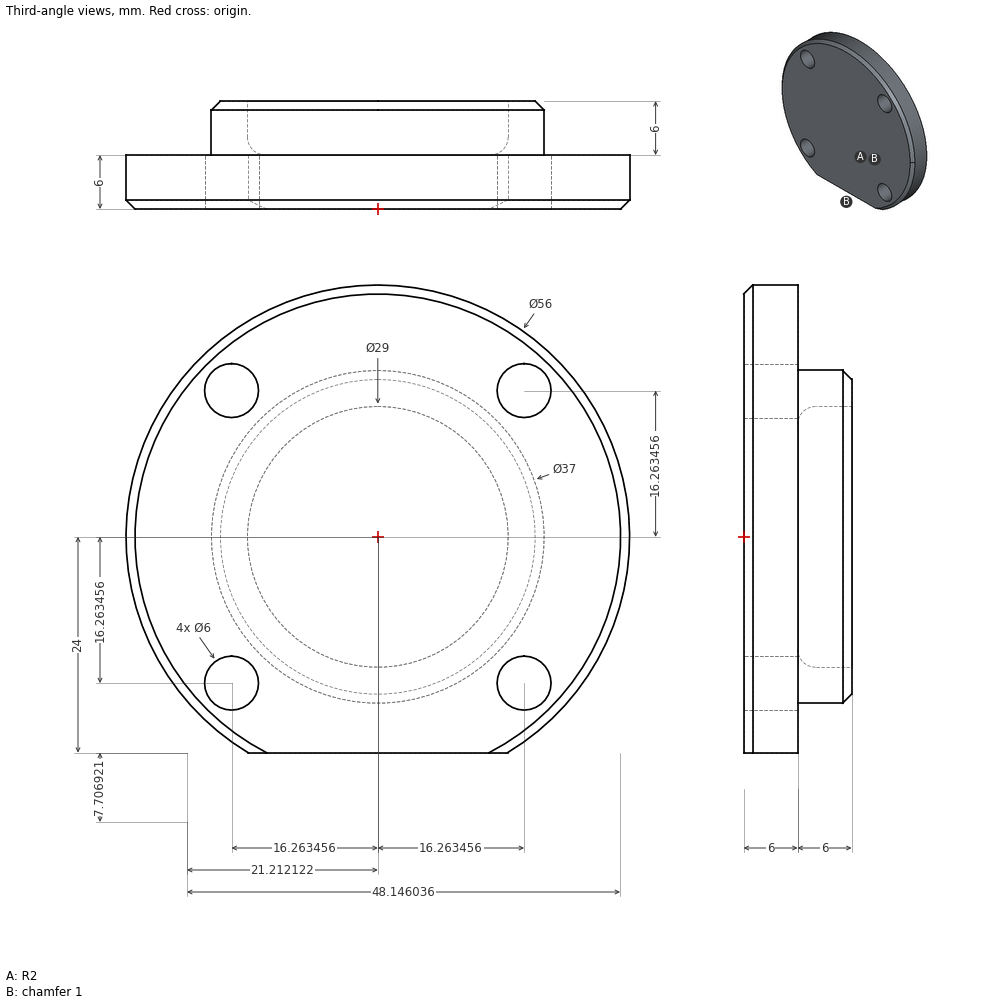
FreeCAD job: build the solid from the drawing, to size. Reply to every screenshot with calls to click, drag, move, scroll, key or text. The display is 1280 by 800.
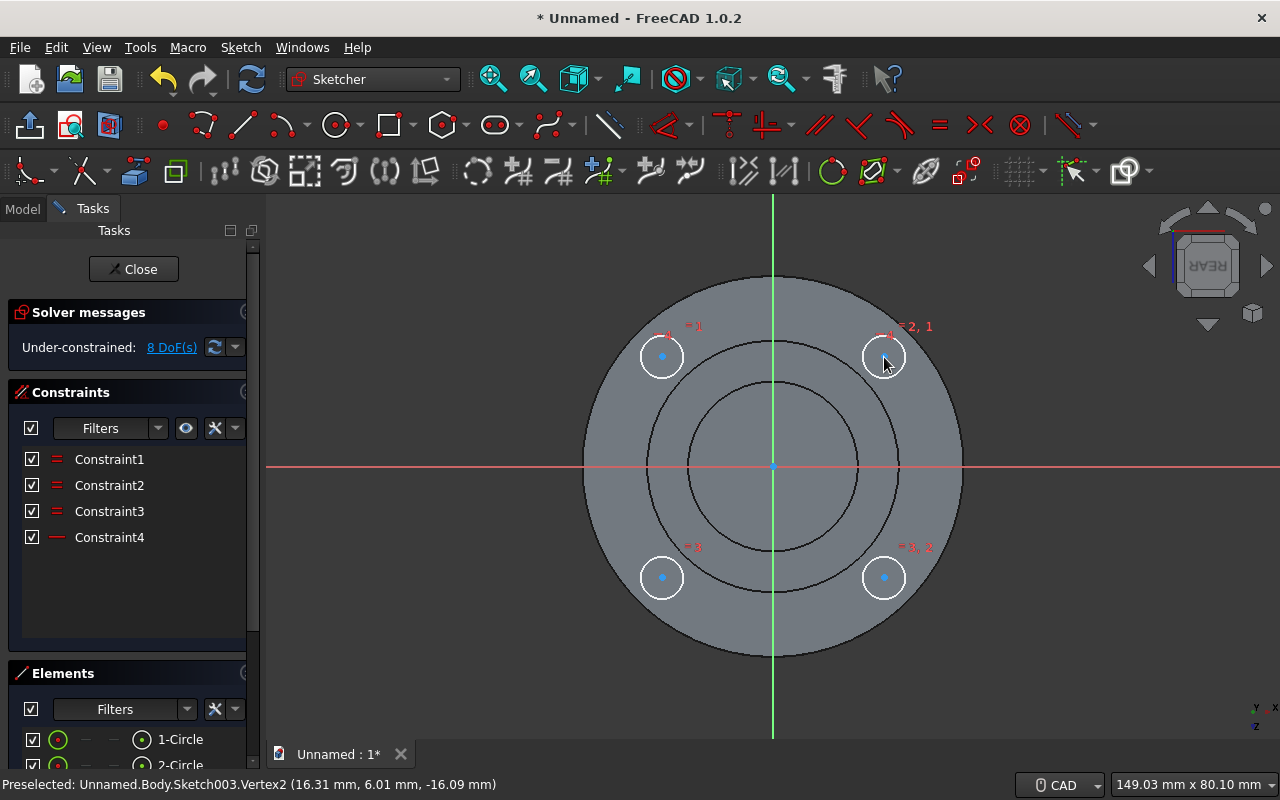
click(884, 357)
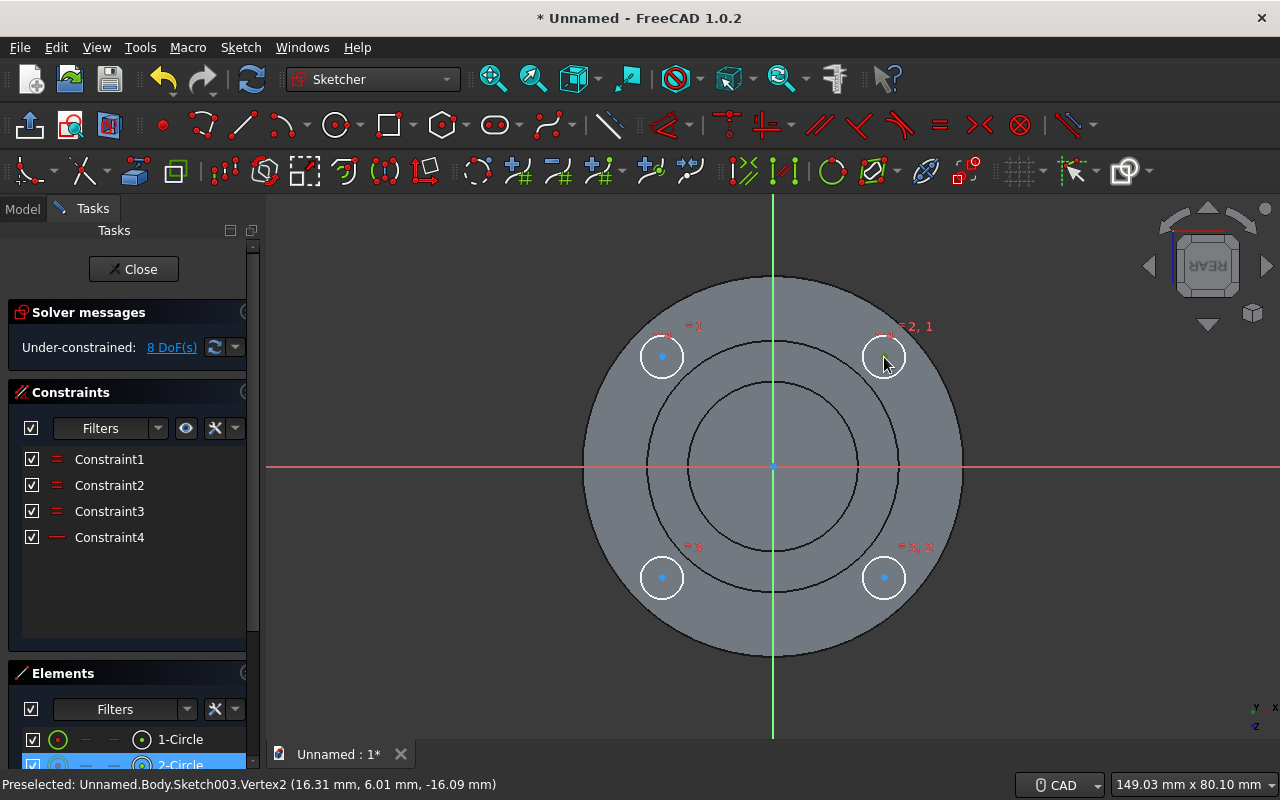
click(884, 578)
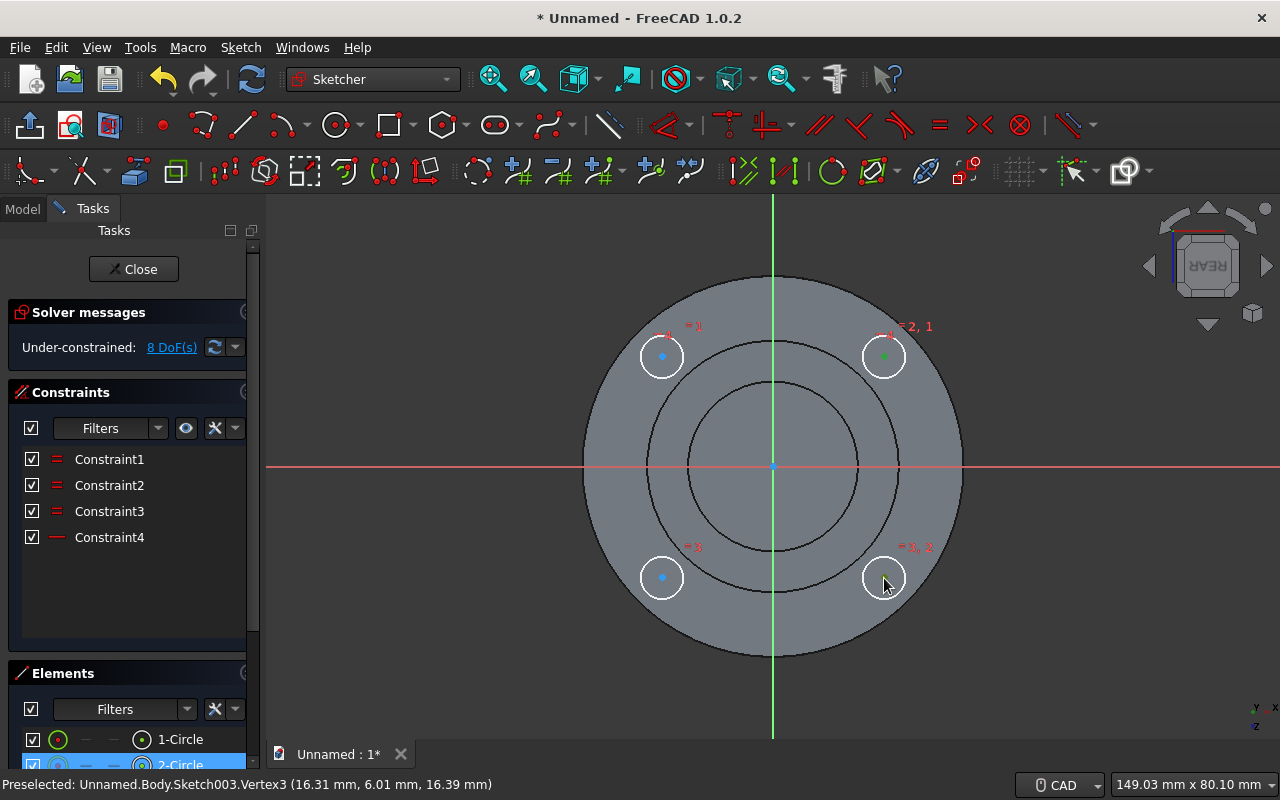
key(v)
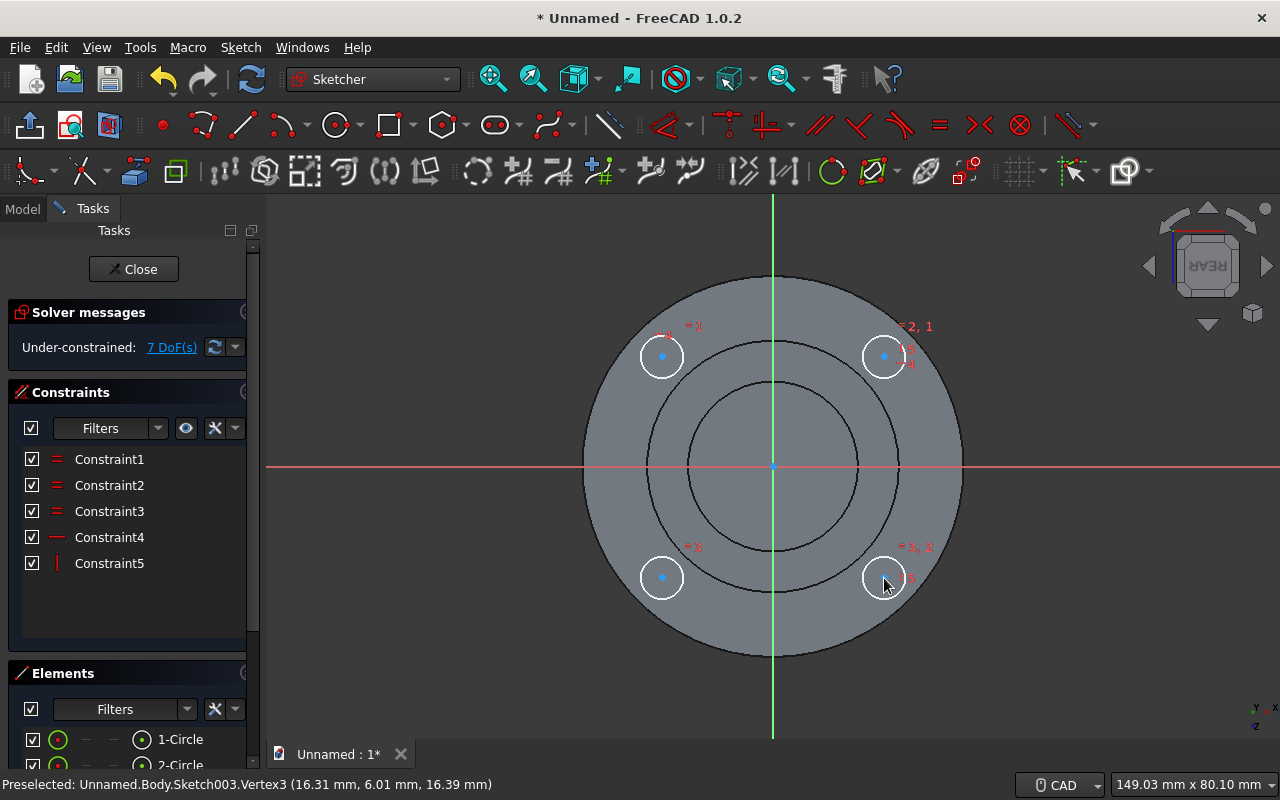
click(662, 357)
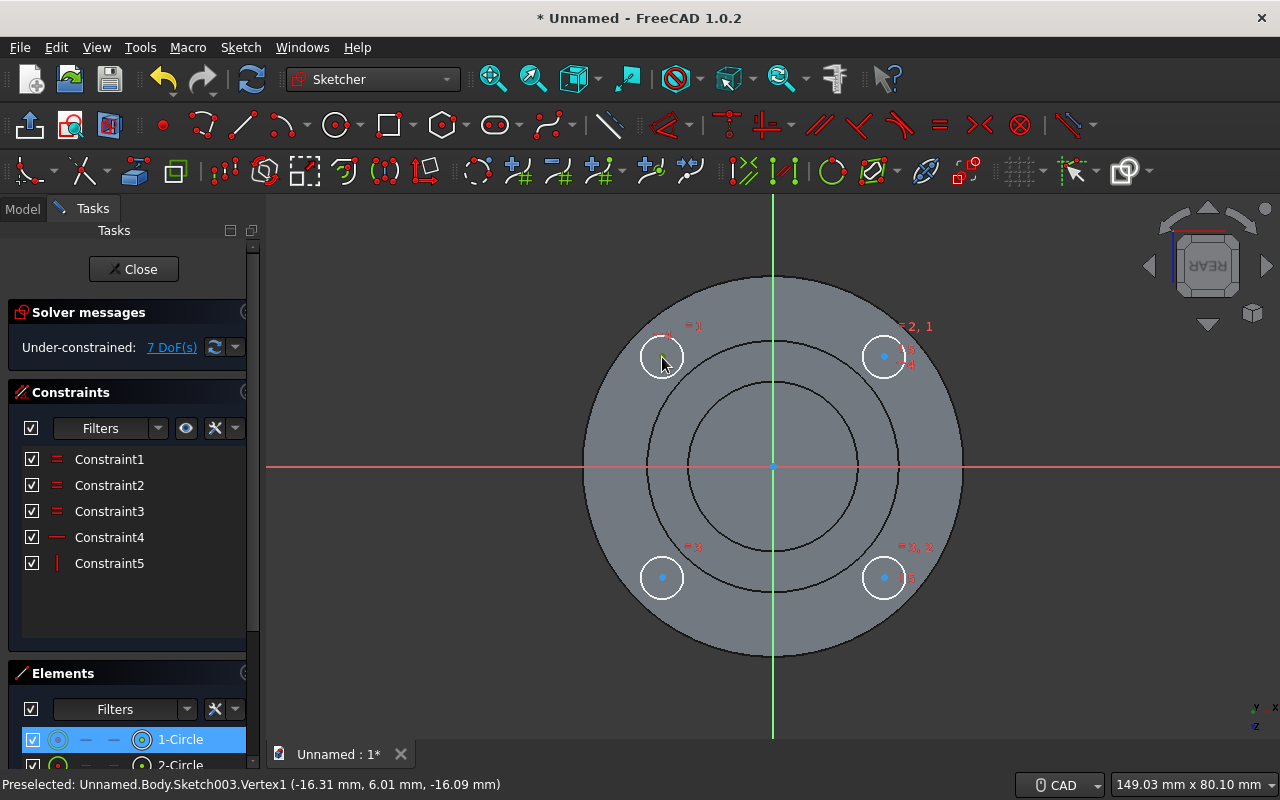
click(662, 578)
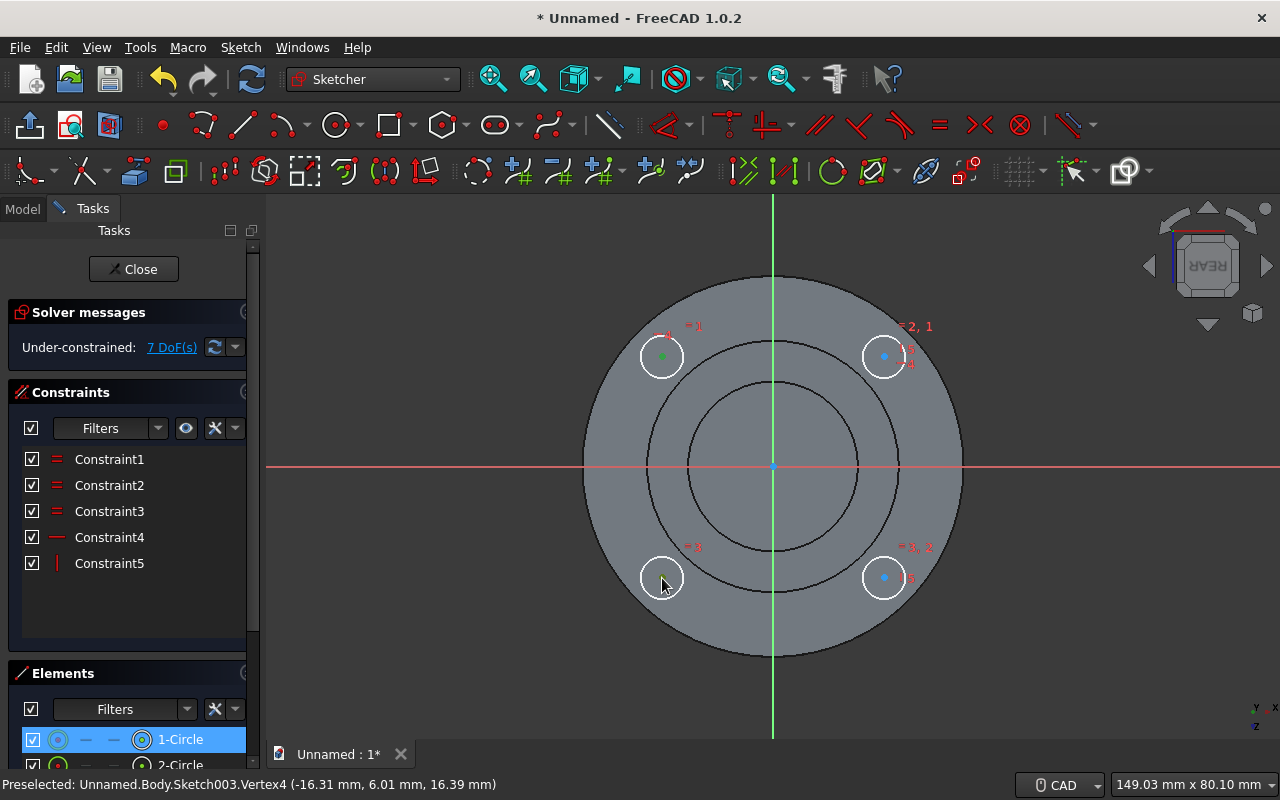
key(v)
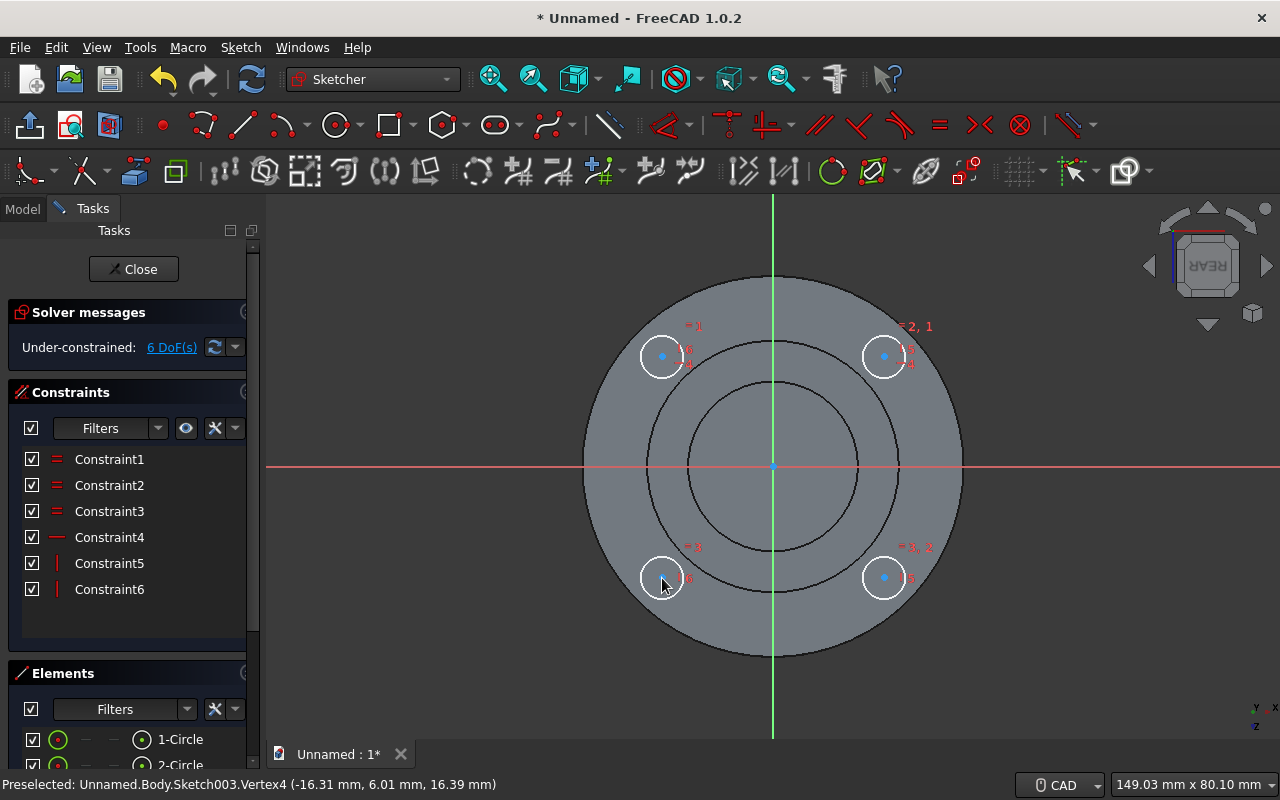
click(884, 578)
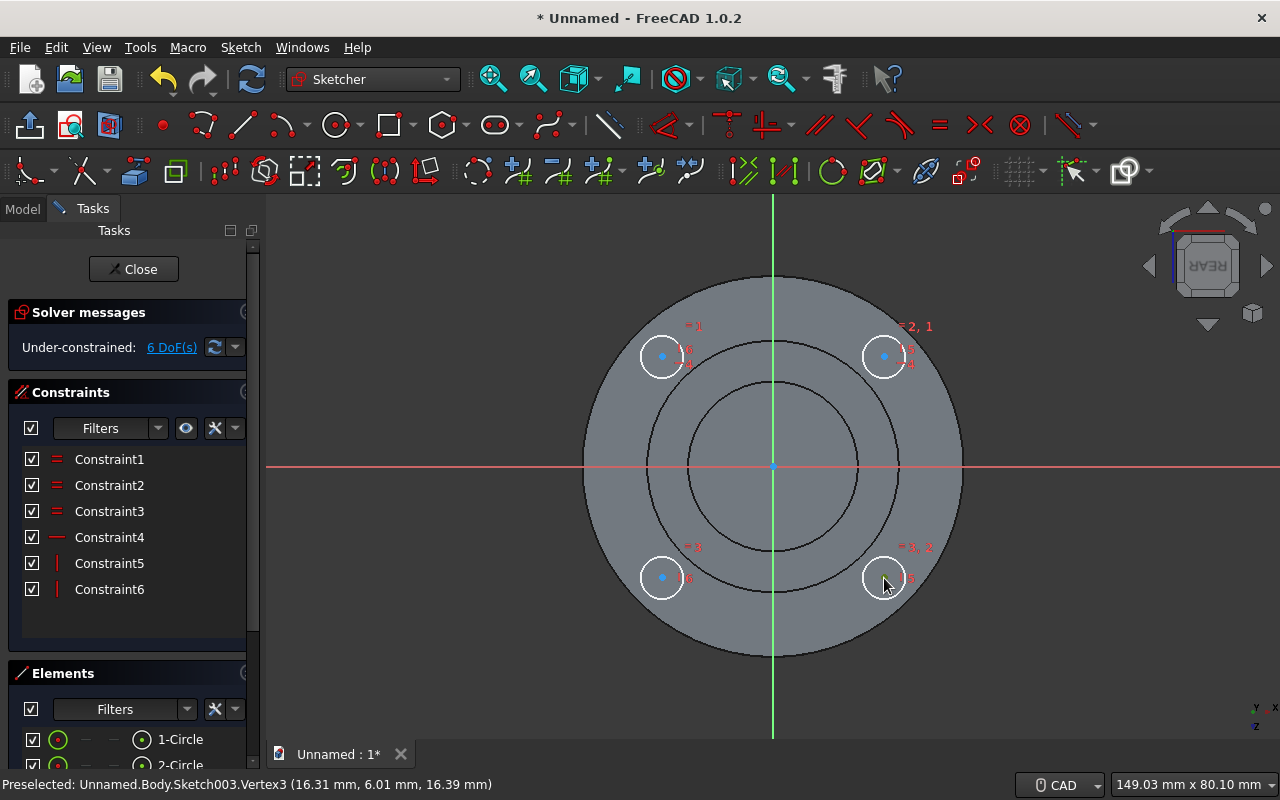
click(662, 578)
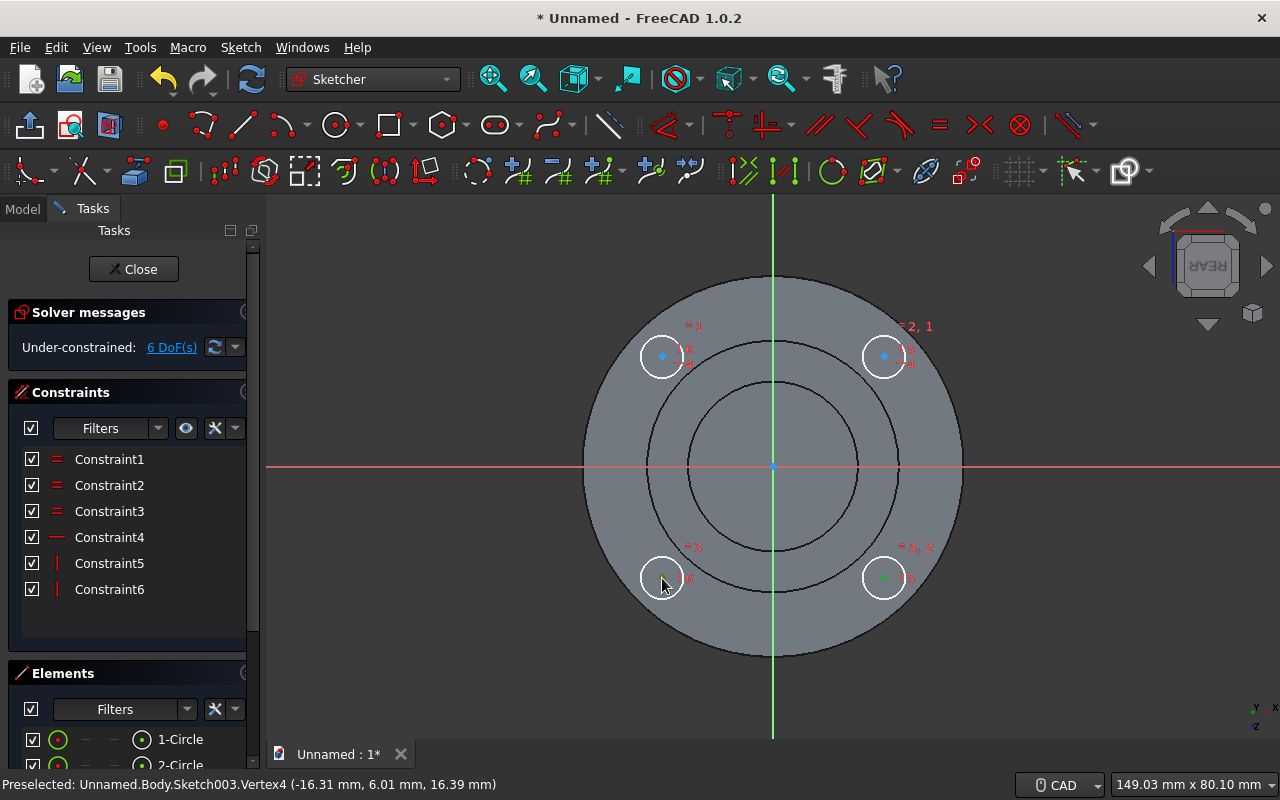
key(h)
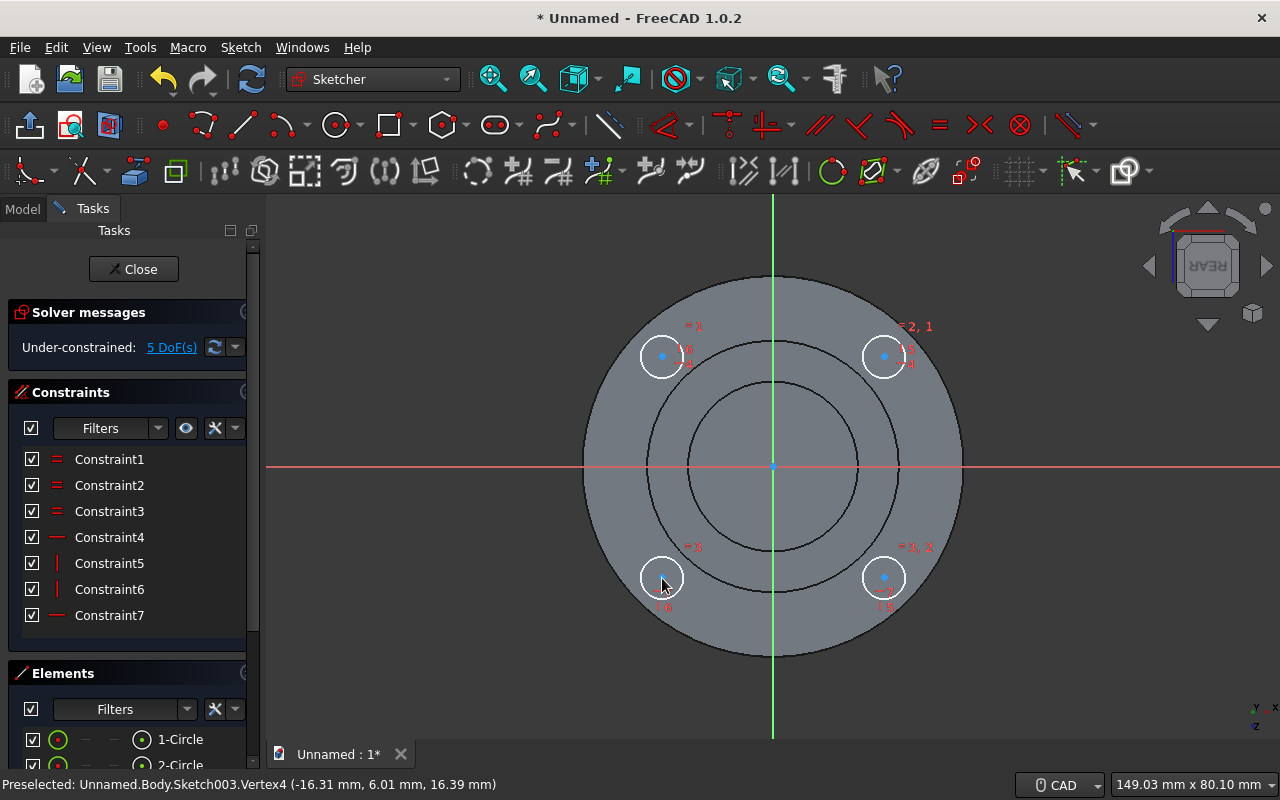
click(664, 126)